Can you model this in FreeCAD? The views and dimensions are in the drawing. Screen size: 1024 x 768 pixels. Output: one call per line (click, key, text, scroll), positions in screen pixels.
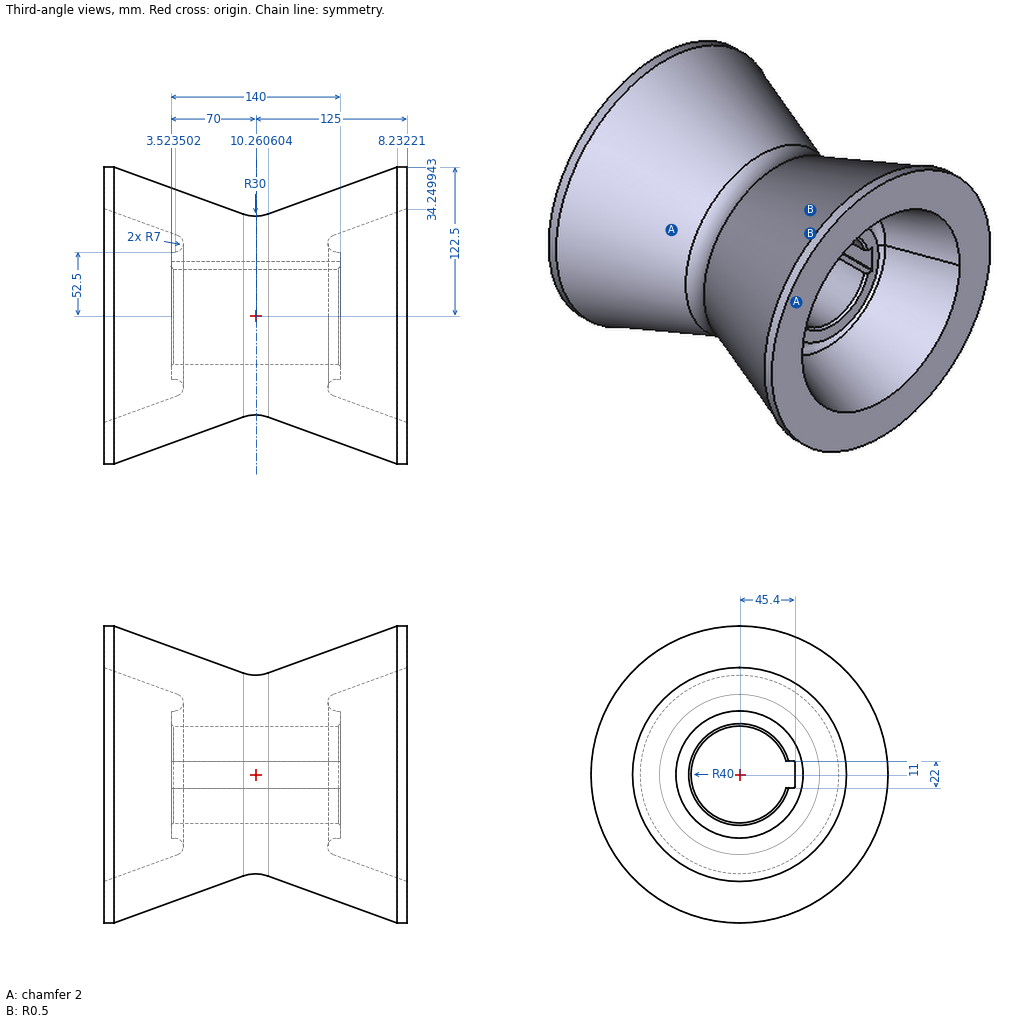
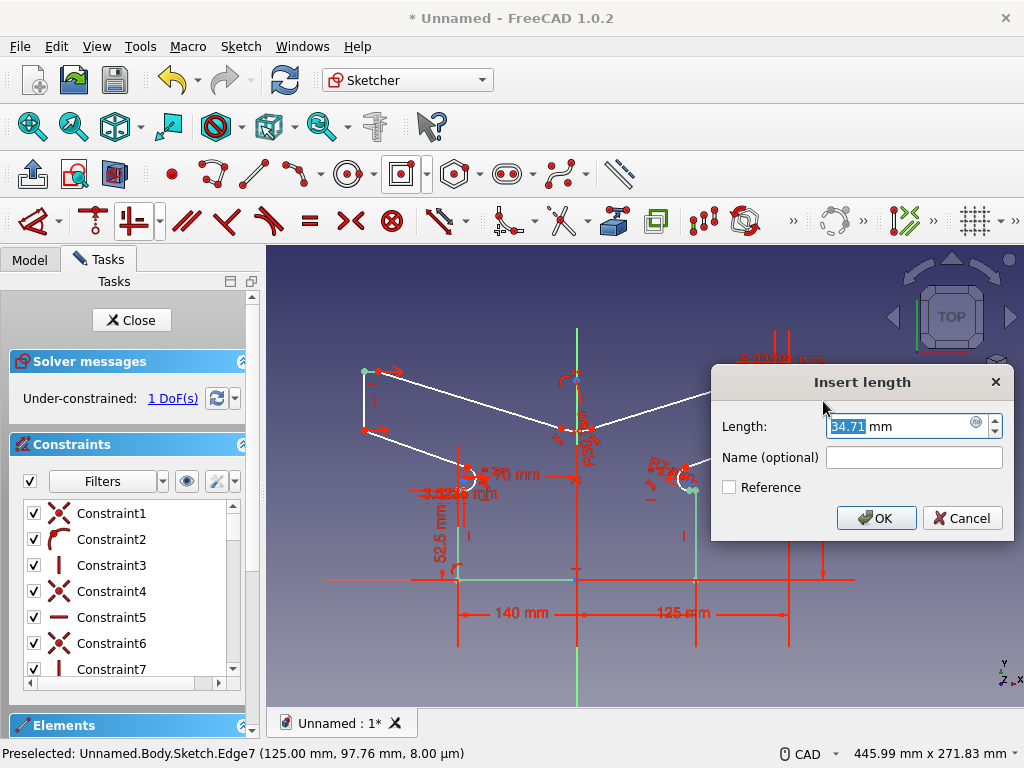
text(34.249943)
key(Return)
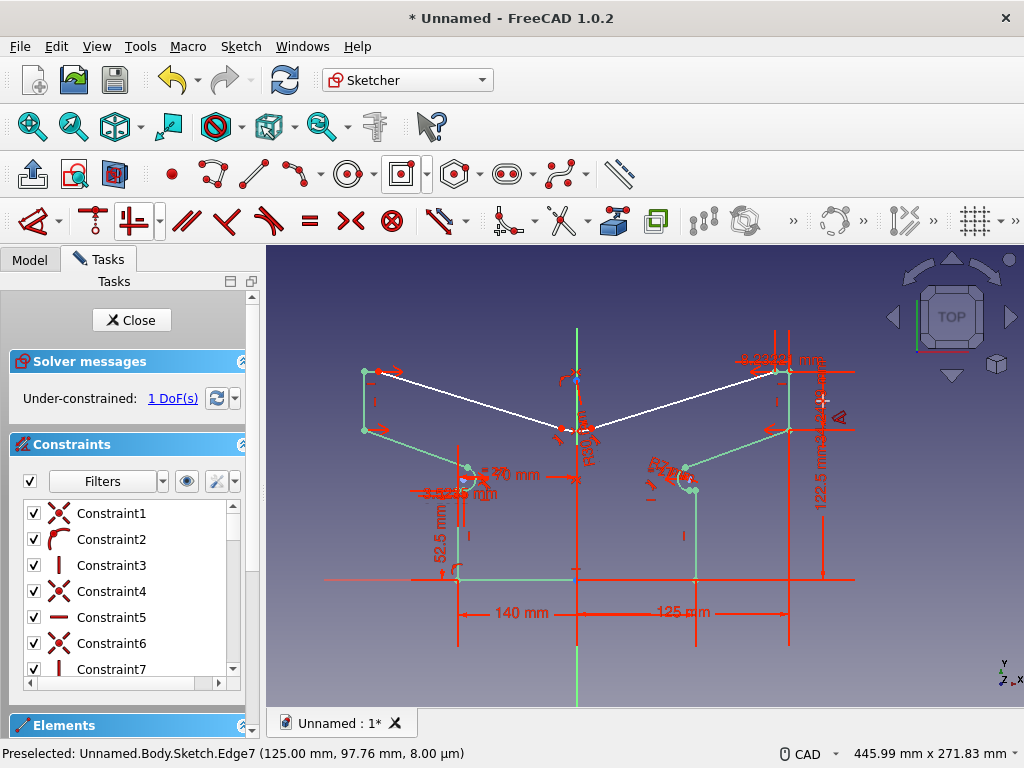
scroll(592, 429, up, 5)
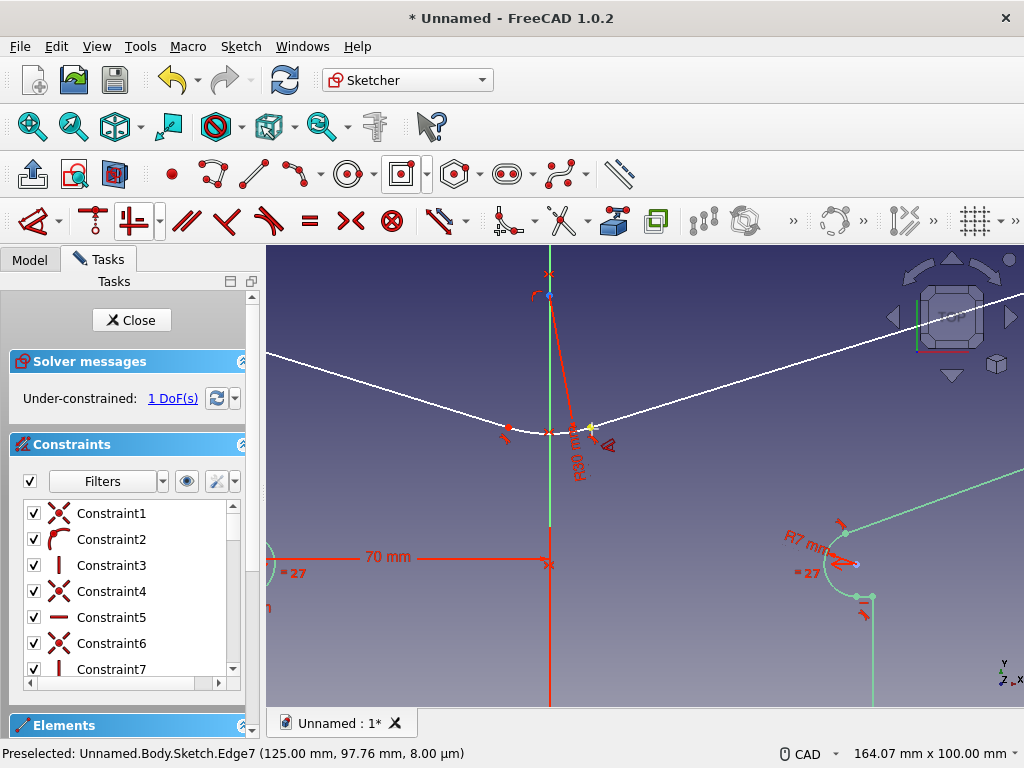
click(591, 428)
click(570, 394)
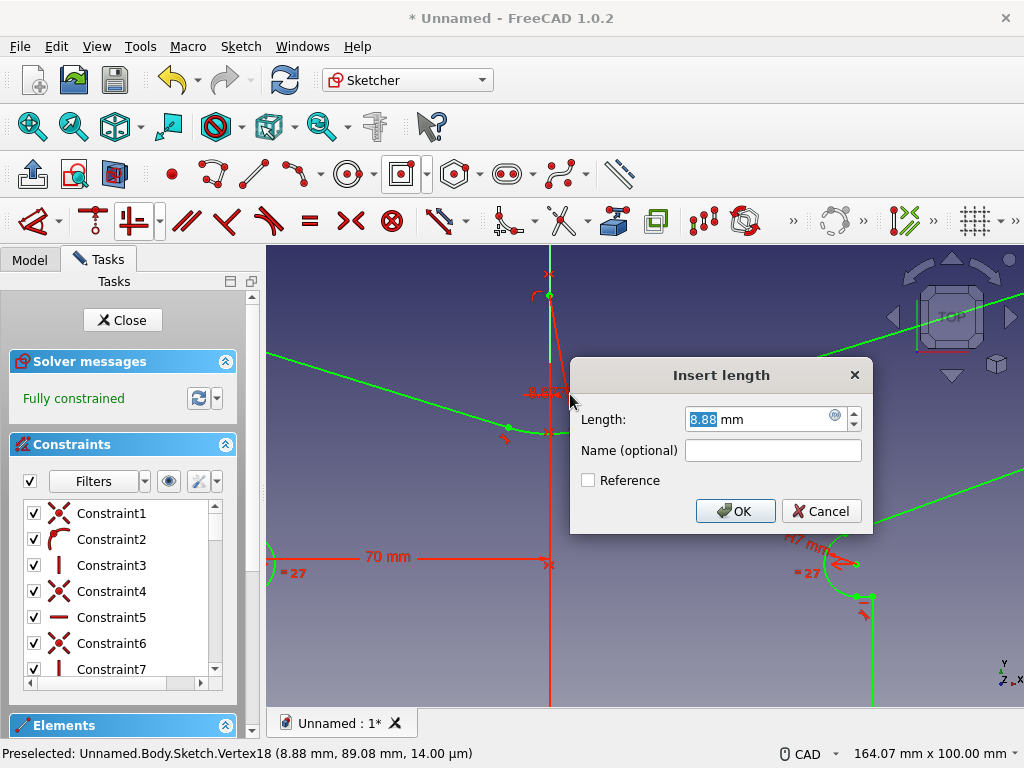
text(10.260604)
key(Return)
key(Escape)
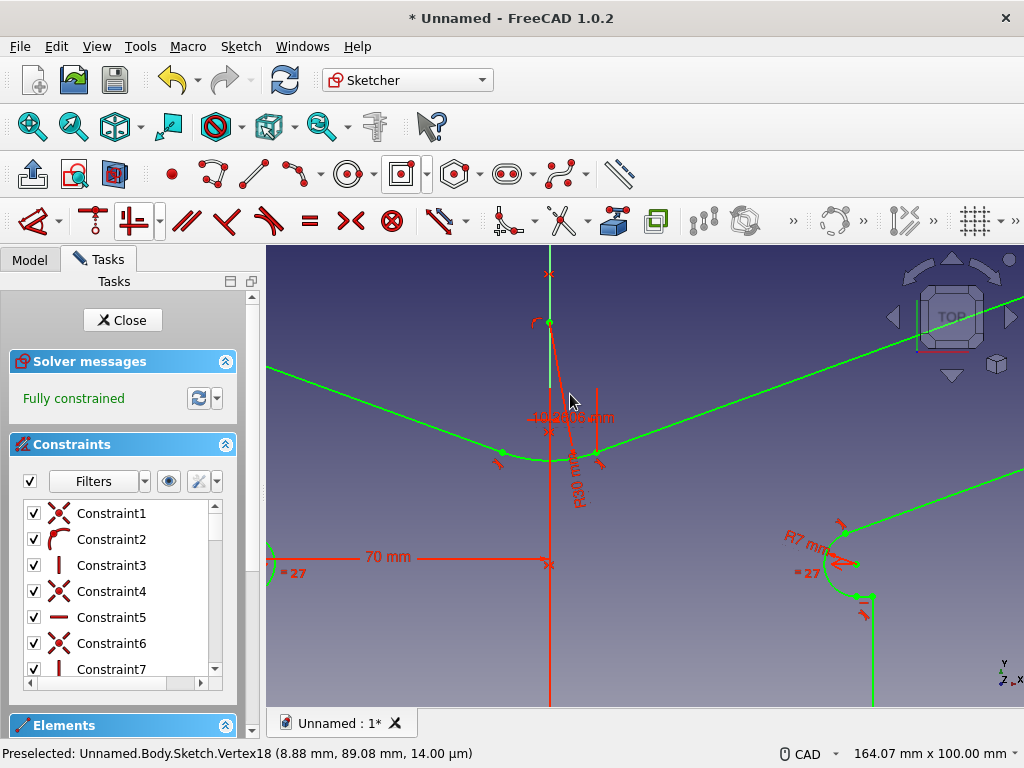
click(123, 320)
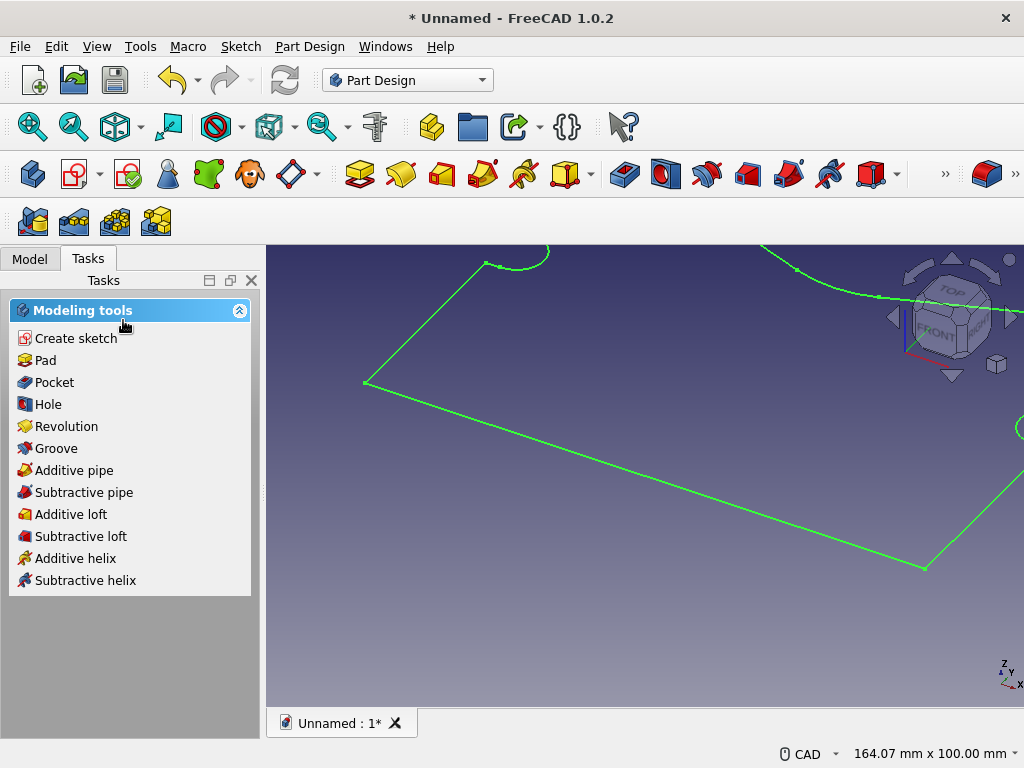
click(401, 174)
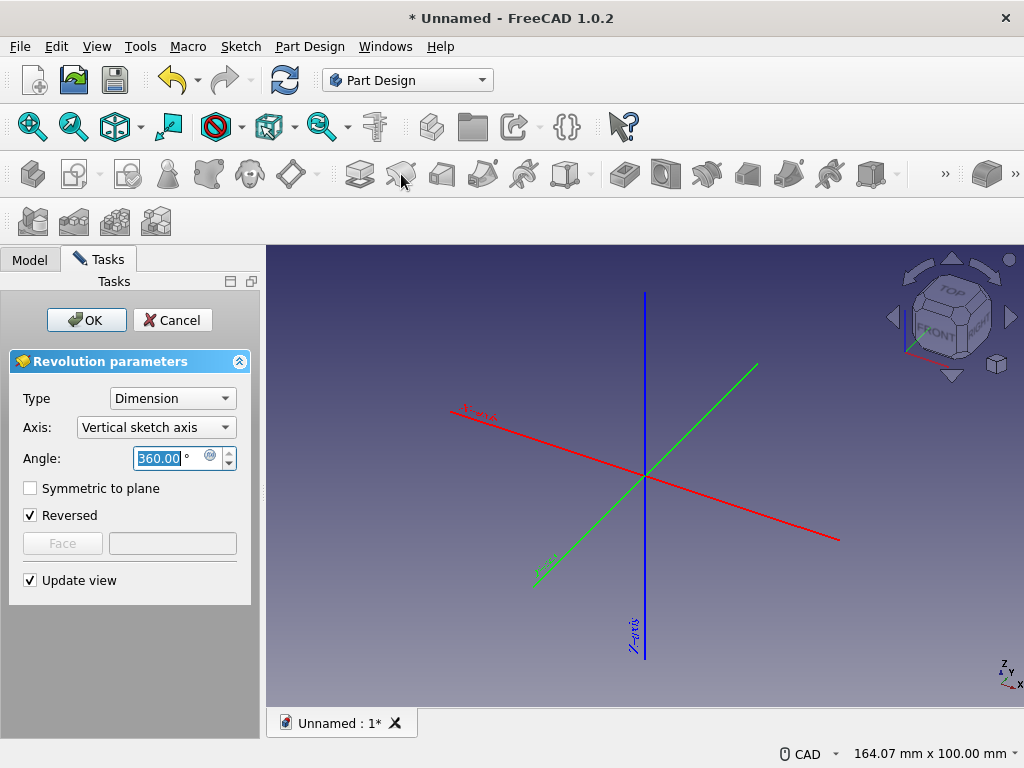
click(157, 428)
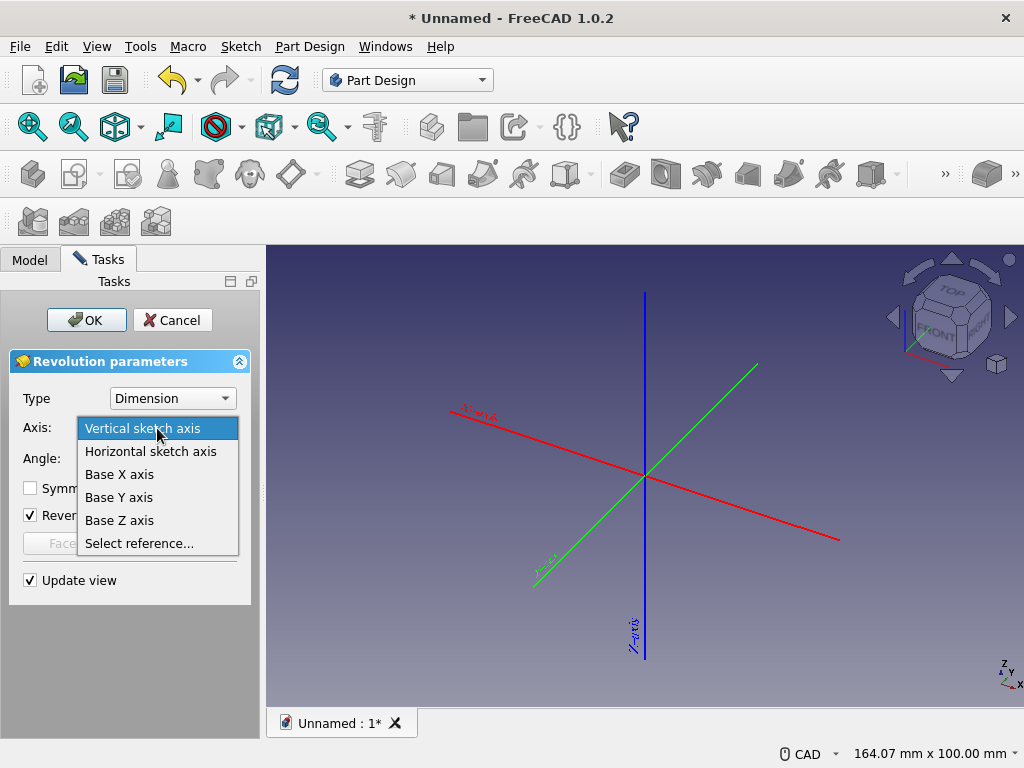
click(156, 452)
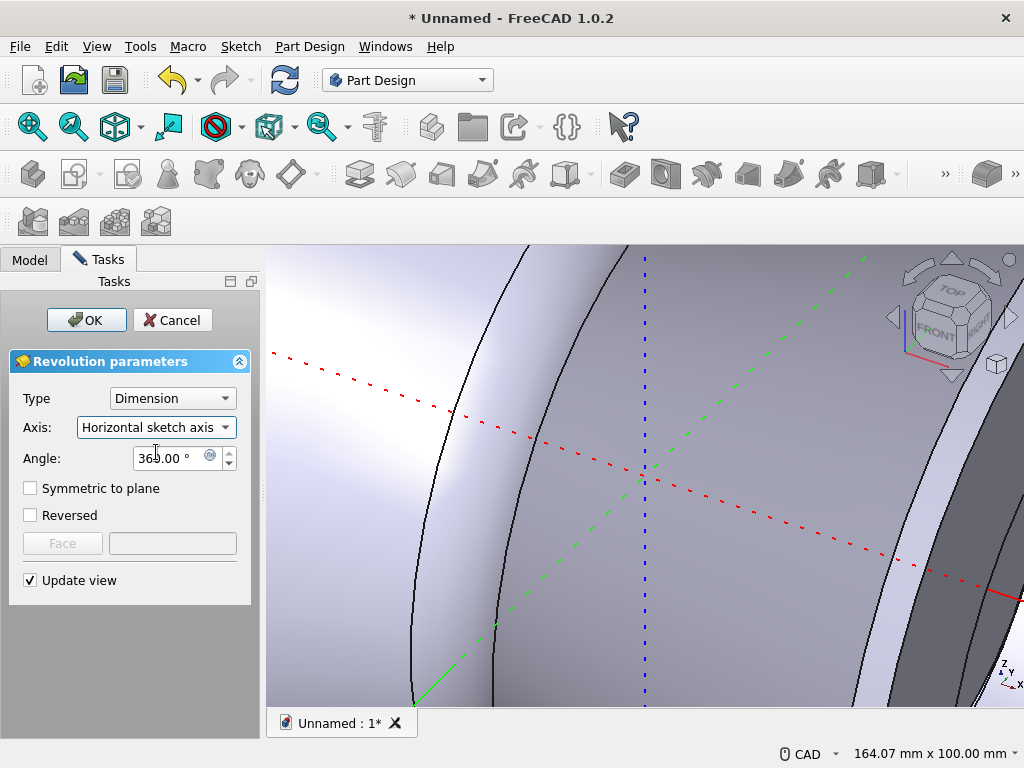
click(87, 320)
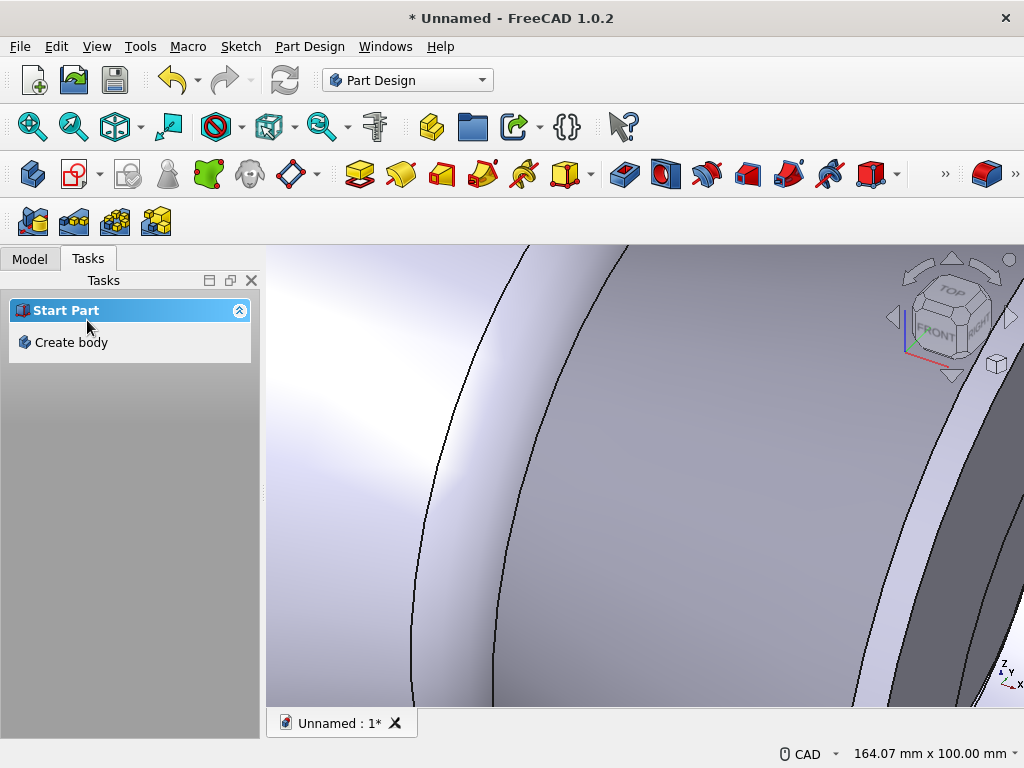
click(33, 128)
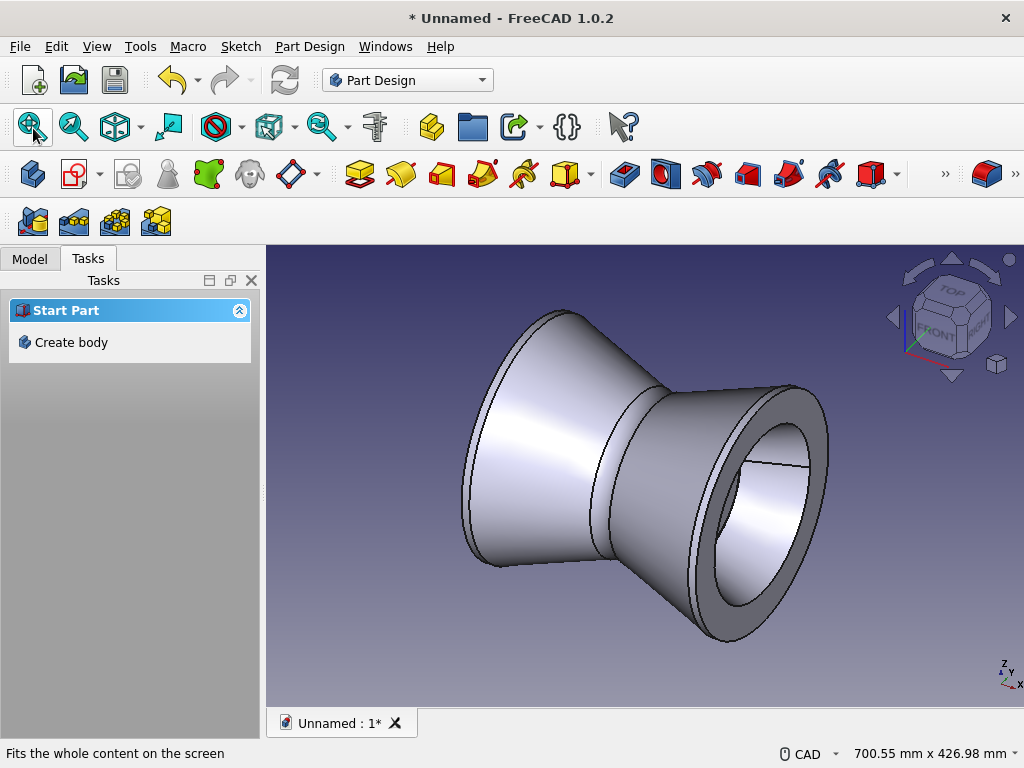
key(6)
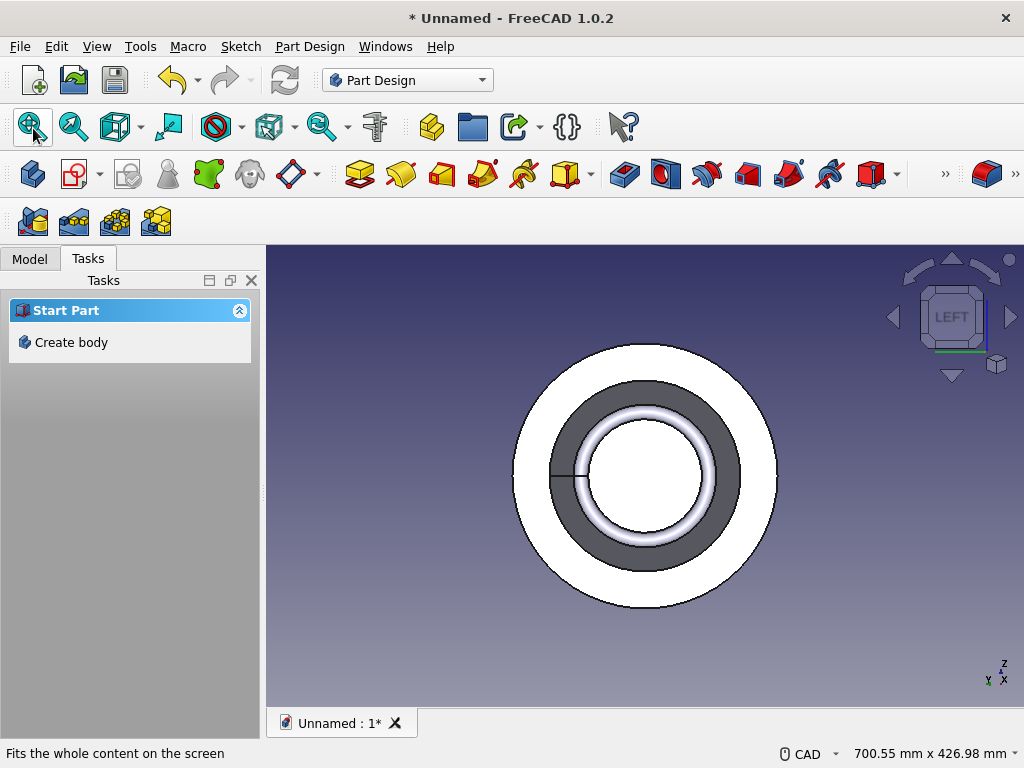
click(645, 475)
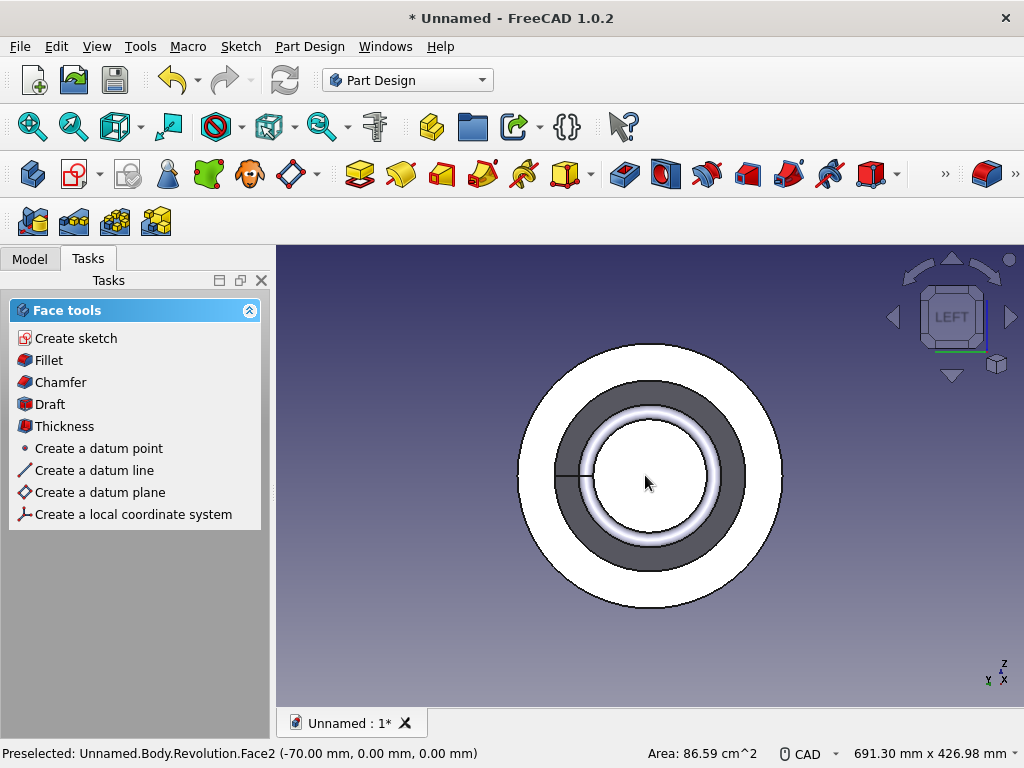
click(74, 174)